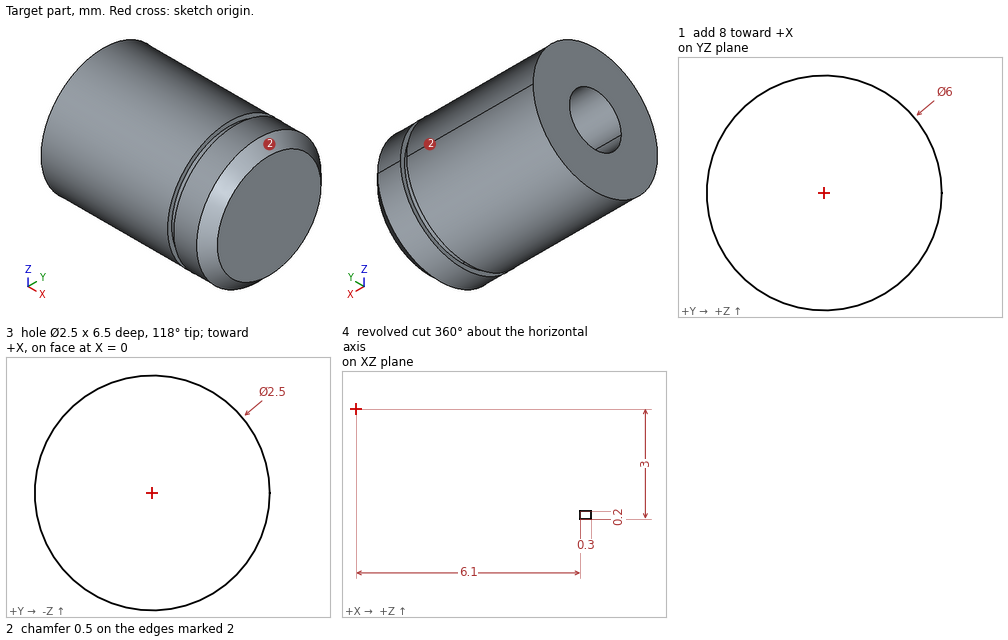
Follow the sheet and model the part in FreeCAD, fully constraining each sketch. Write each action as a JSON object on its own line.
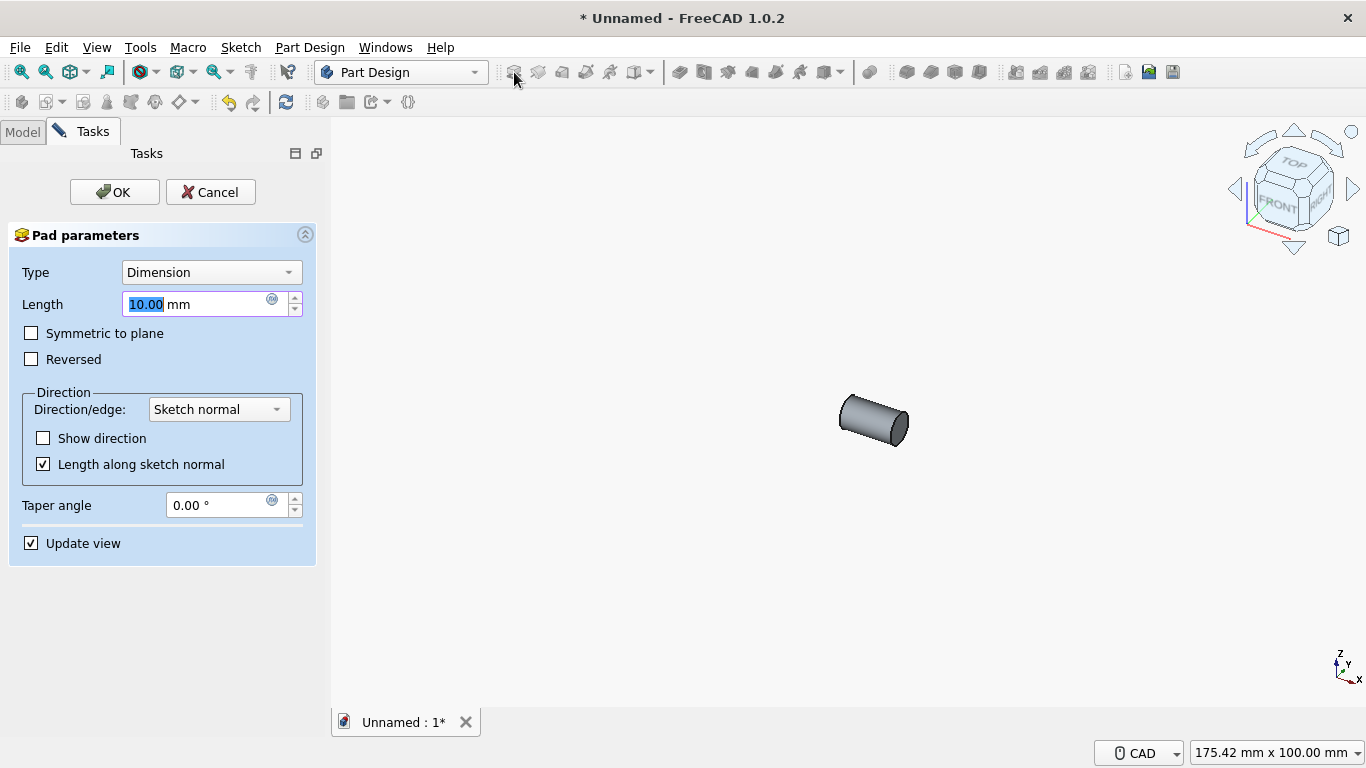
{"action": "type", "text": "8"}
{"action": "key", "text": "Tab"}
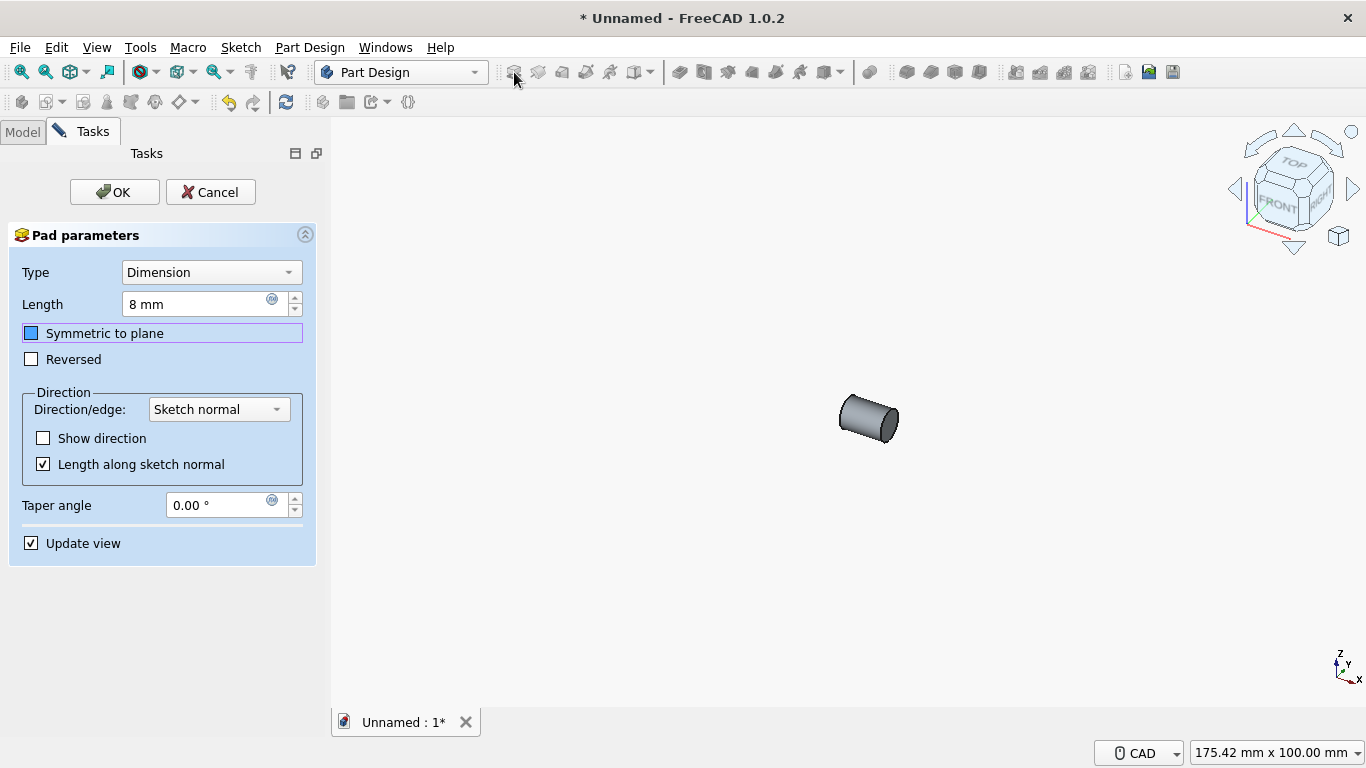
{"action": "left_click", "coordinate": [115, 192]}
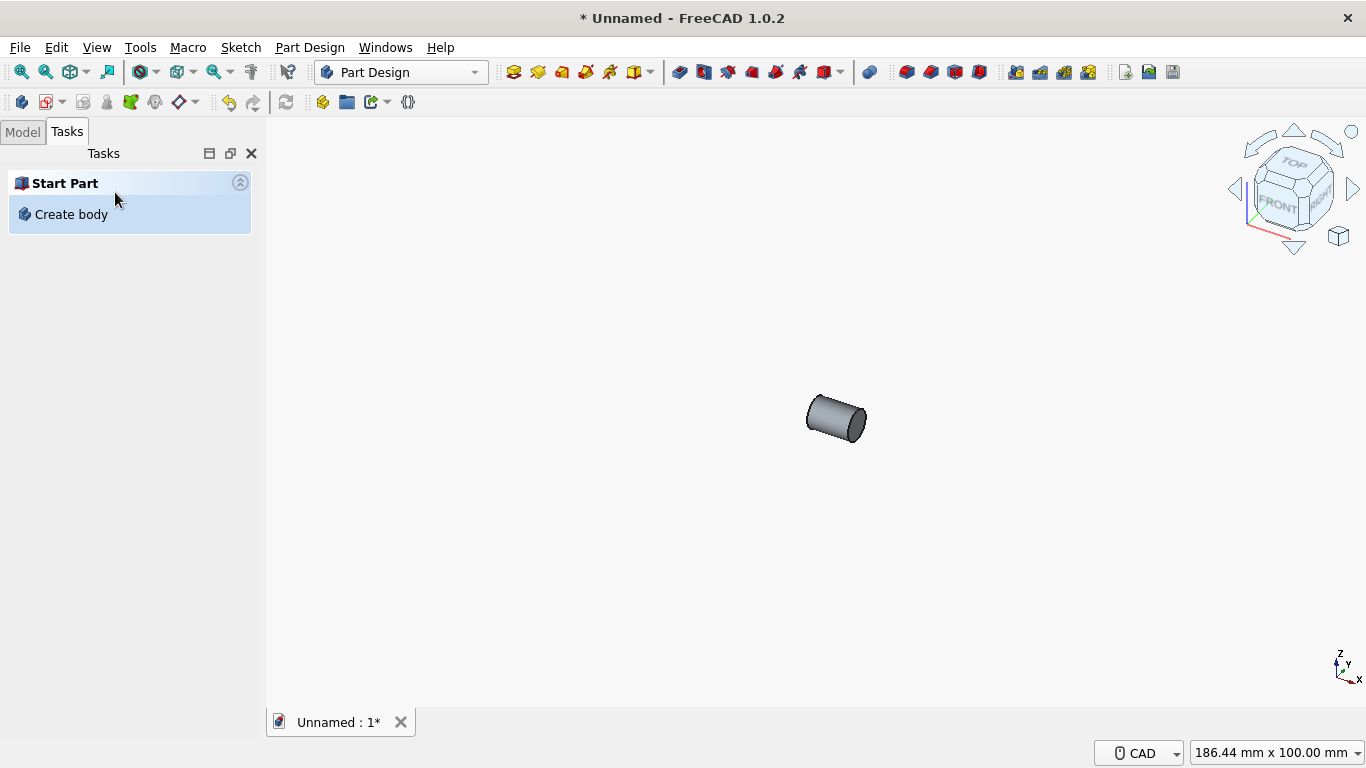
{"action": "left_click", "coordinate": [22, 72]}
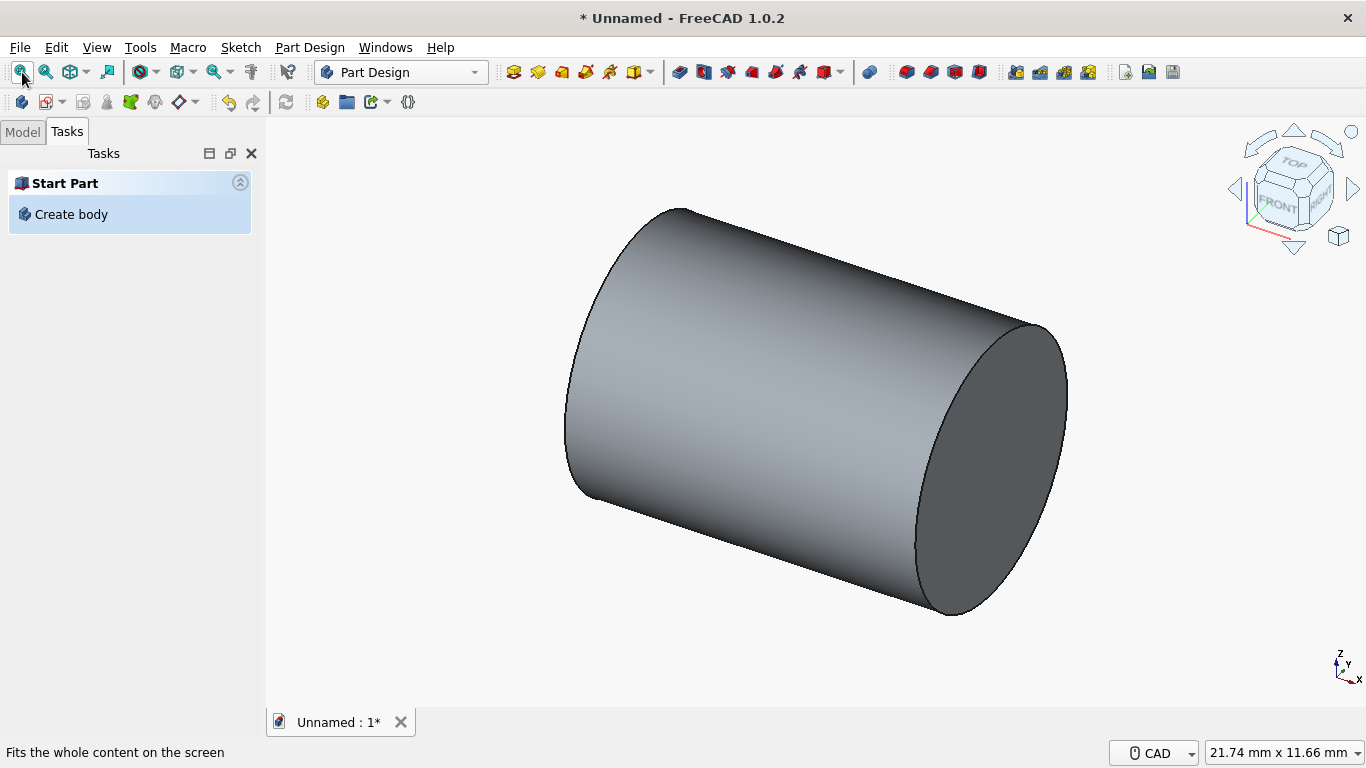
{"action": "left_click", "coordinate": [915, 544]}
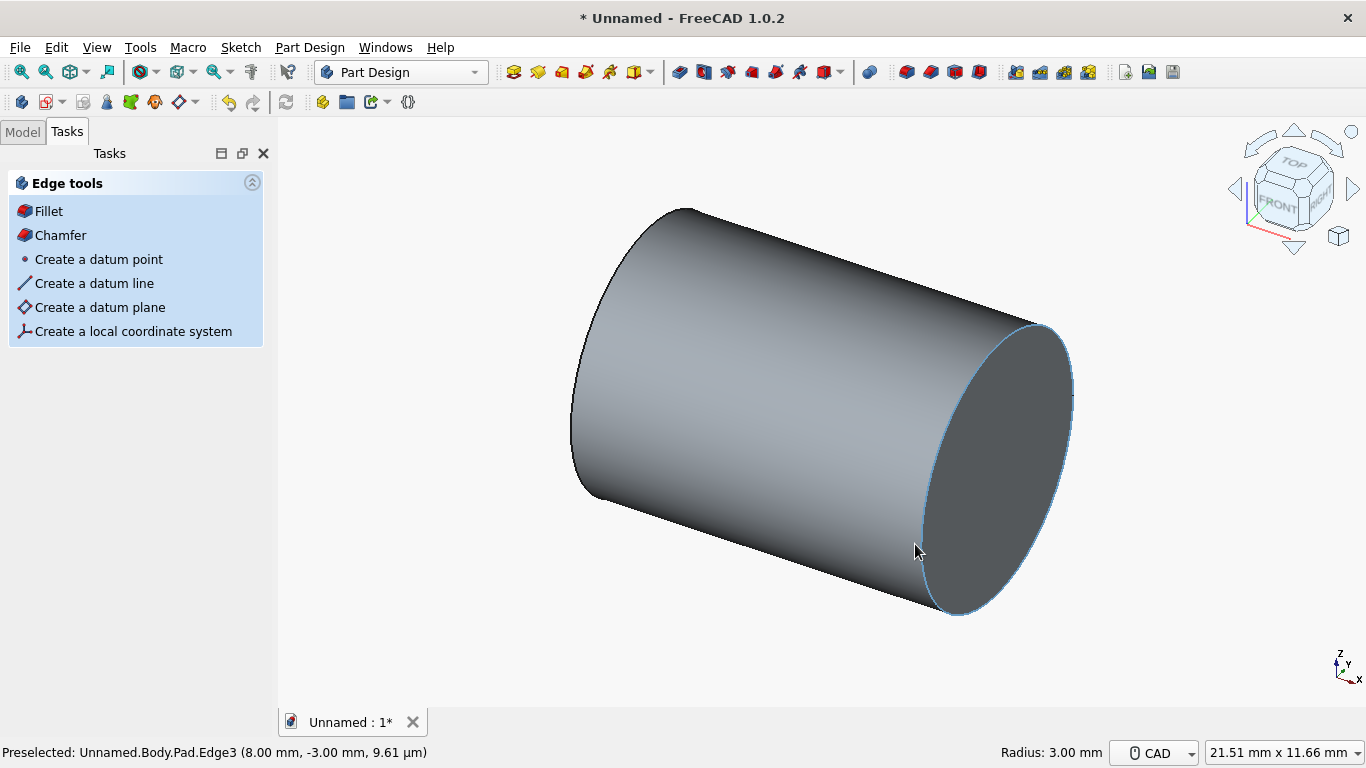
{"action": "left_click", "coordinate": [932, 72]}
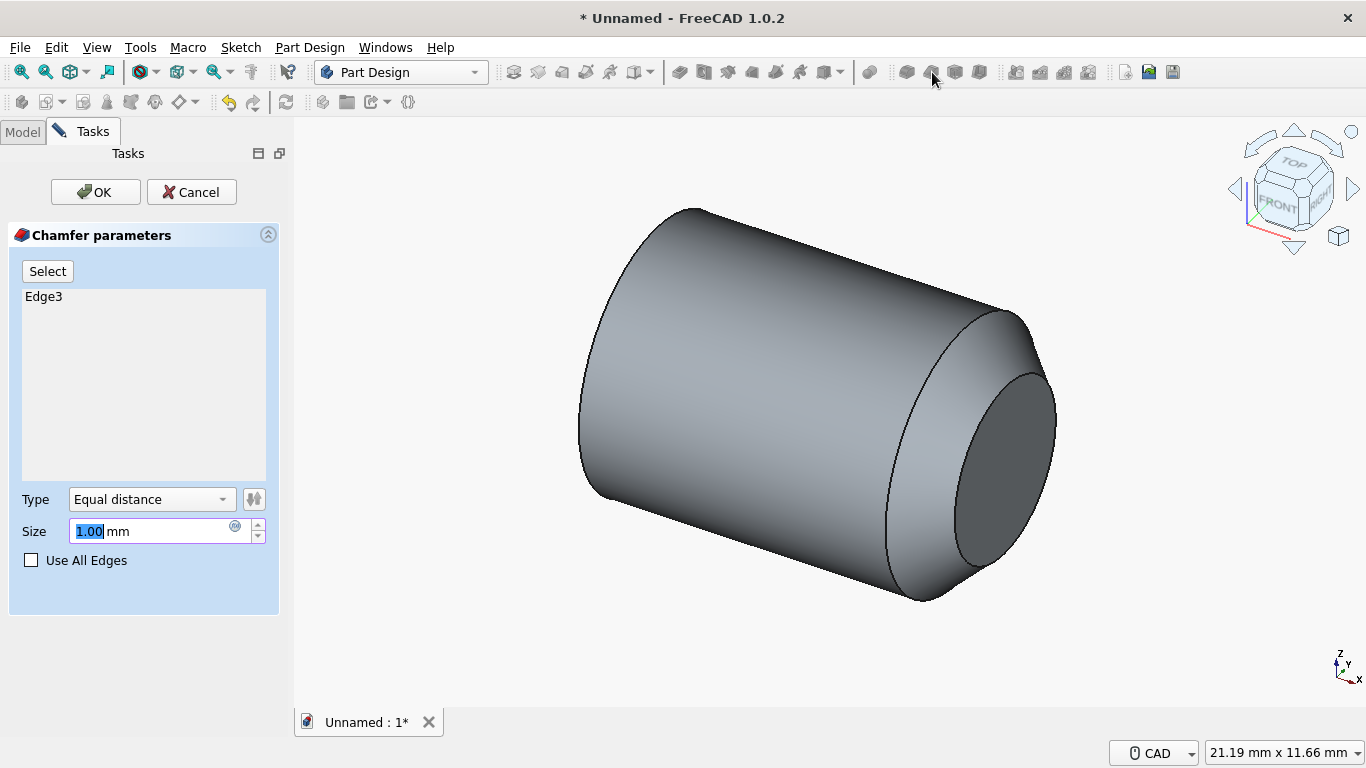
{"action": "type", "text": "0.5"}
{"action": "key", "text": "Tab"}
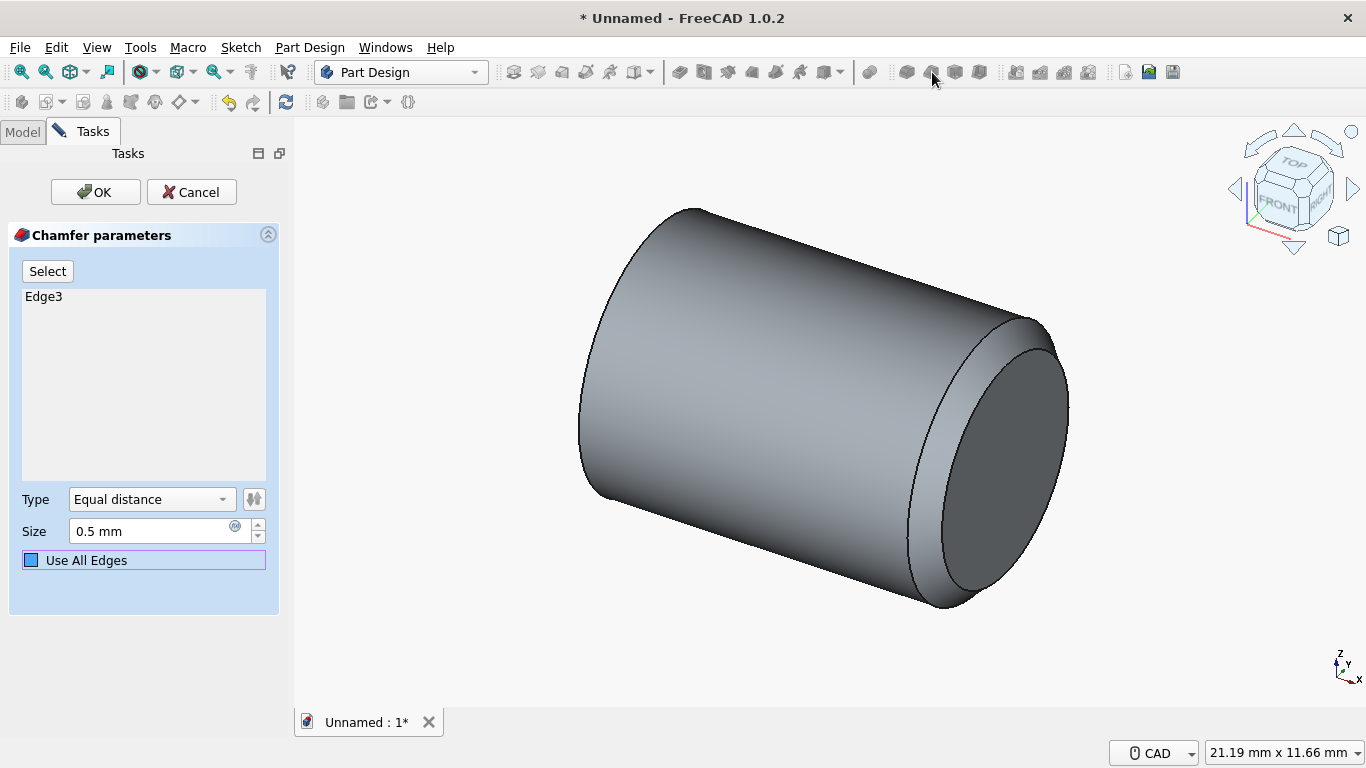
{"action": "left_click", "coordinate": [96, 192]}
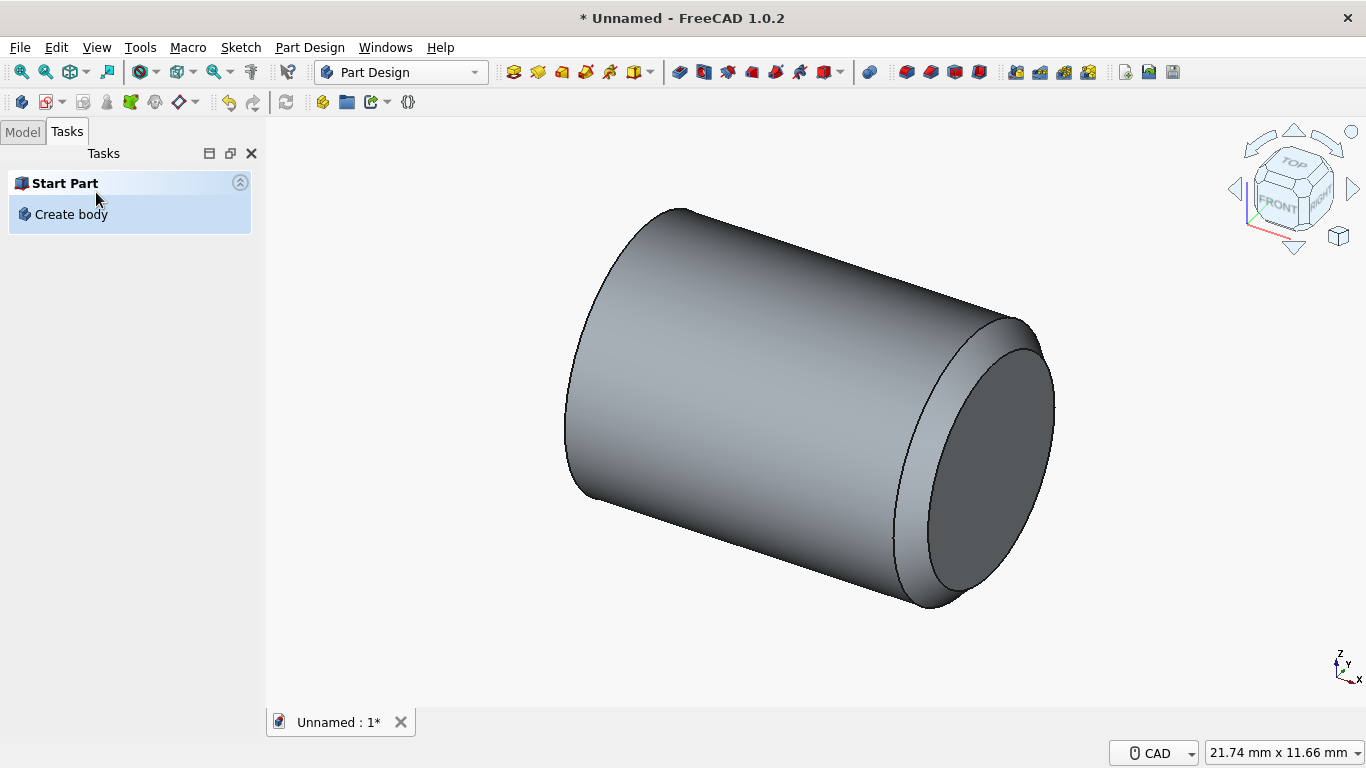
{"action": "key", "text": "6"}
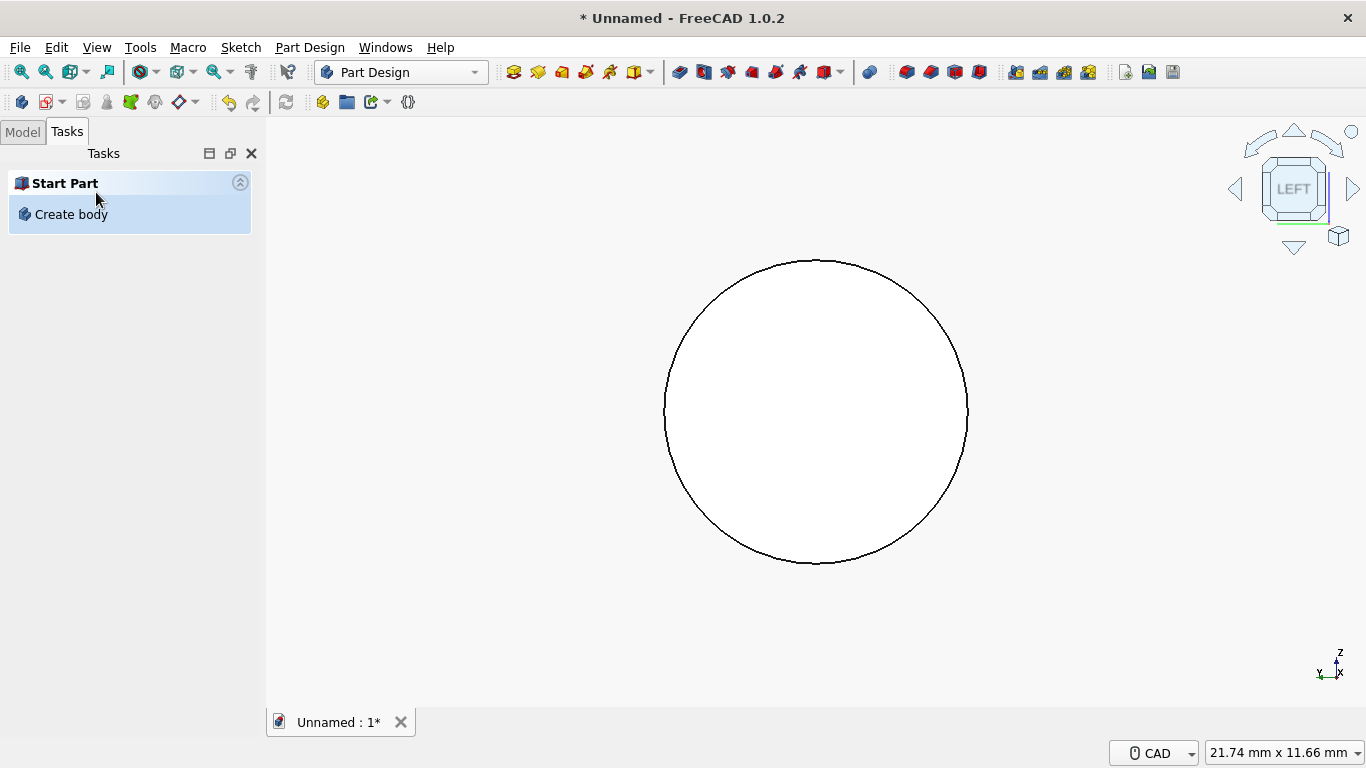
{"action": "left_click", "coordinate": [816, 411]}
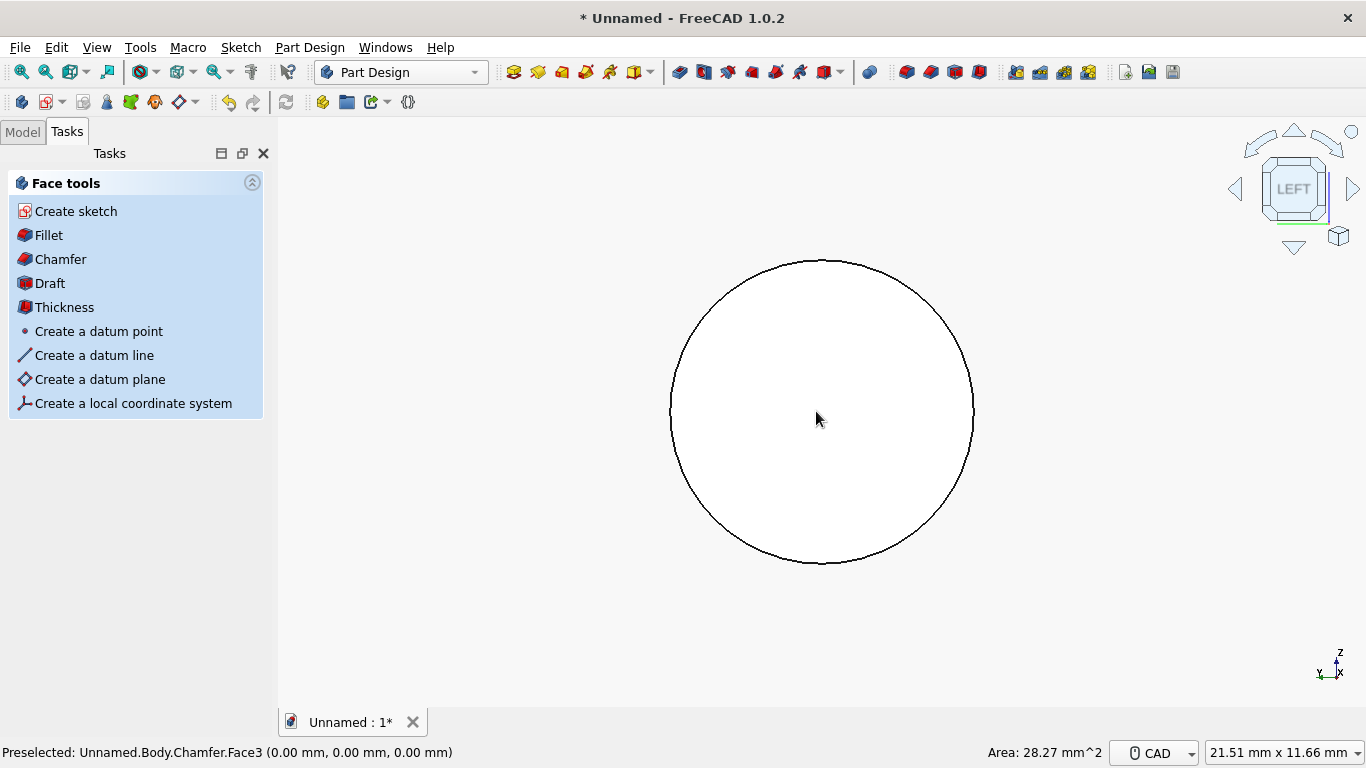
{"action": "left_click", "coordinate": [46, 102]}